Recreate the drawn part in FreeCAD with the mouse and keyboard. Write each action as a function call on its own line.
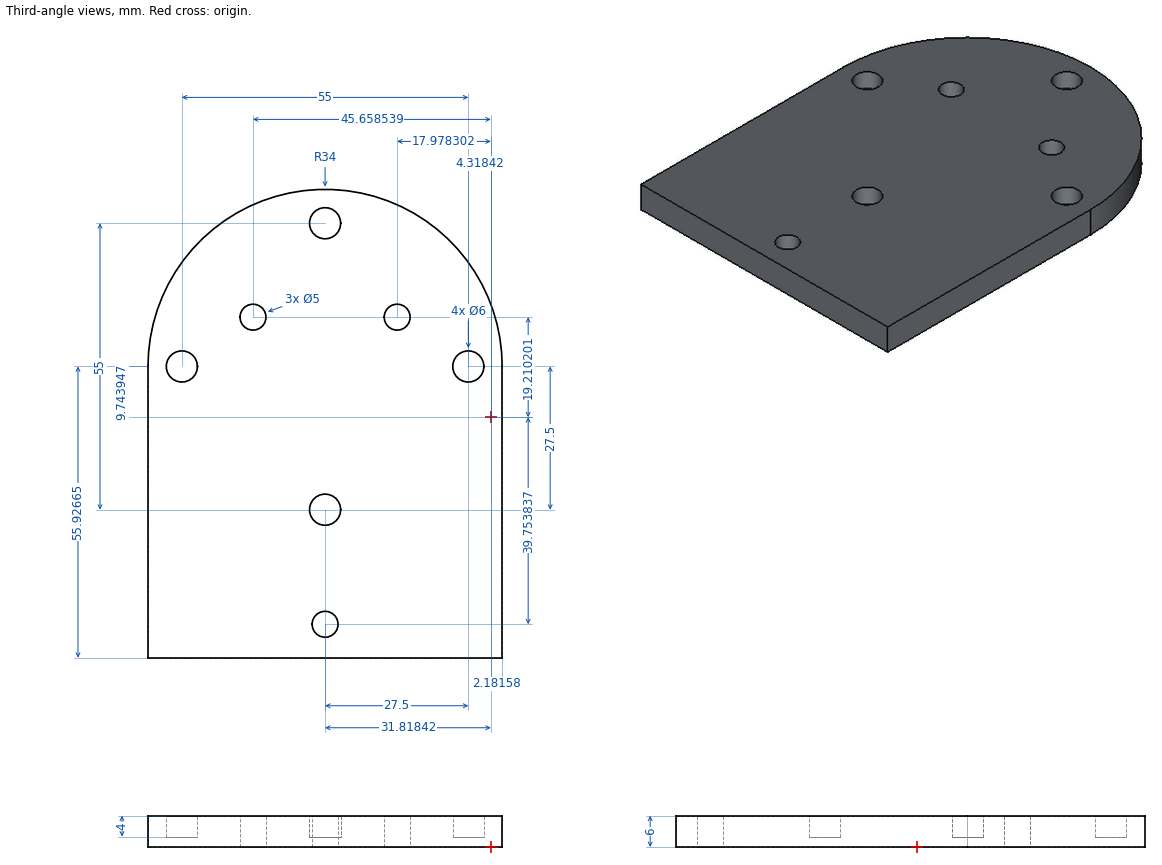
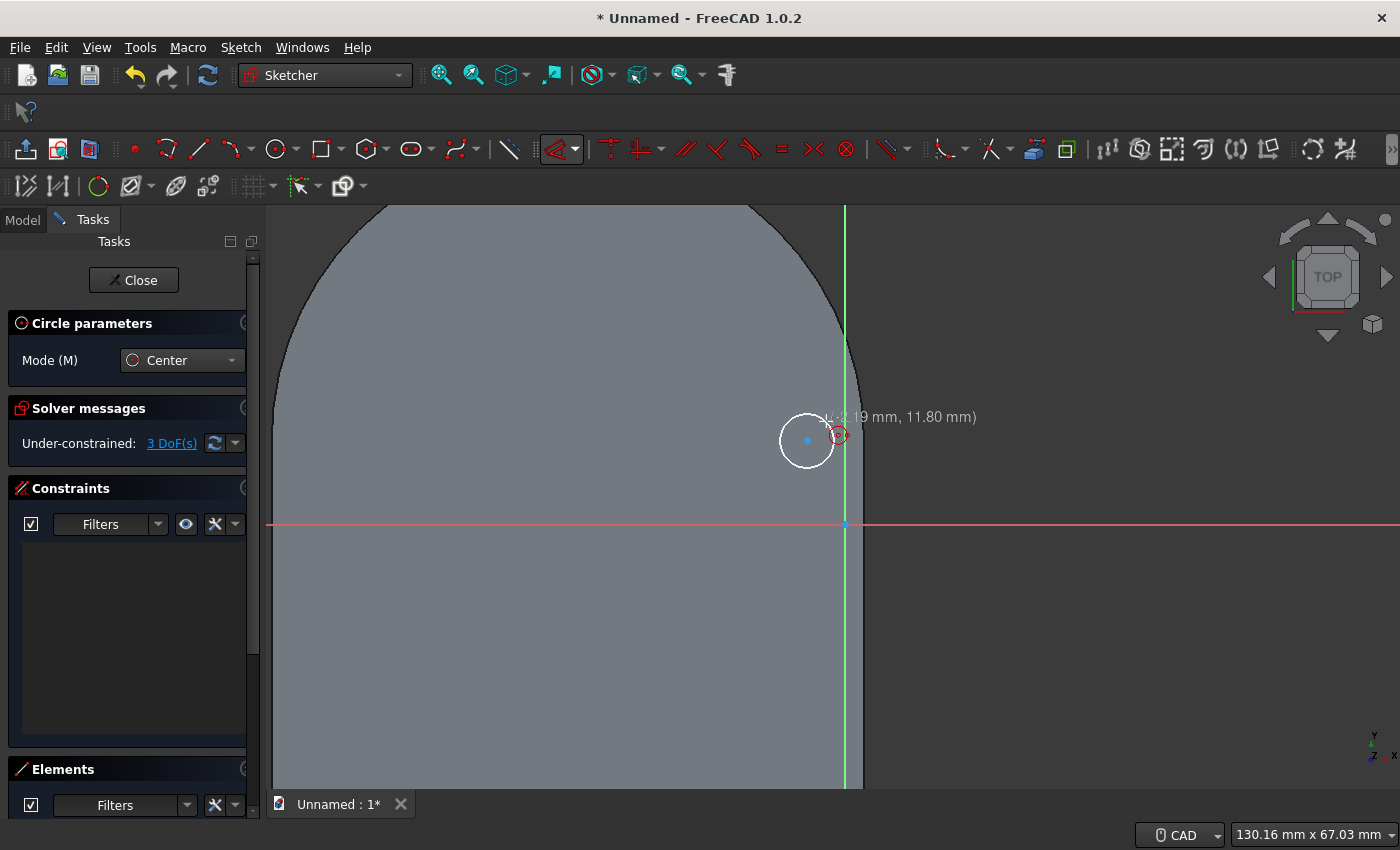
click(568, 680)
click(586, 661)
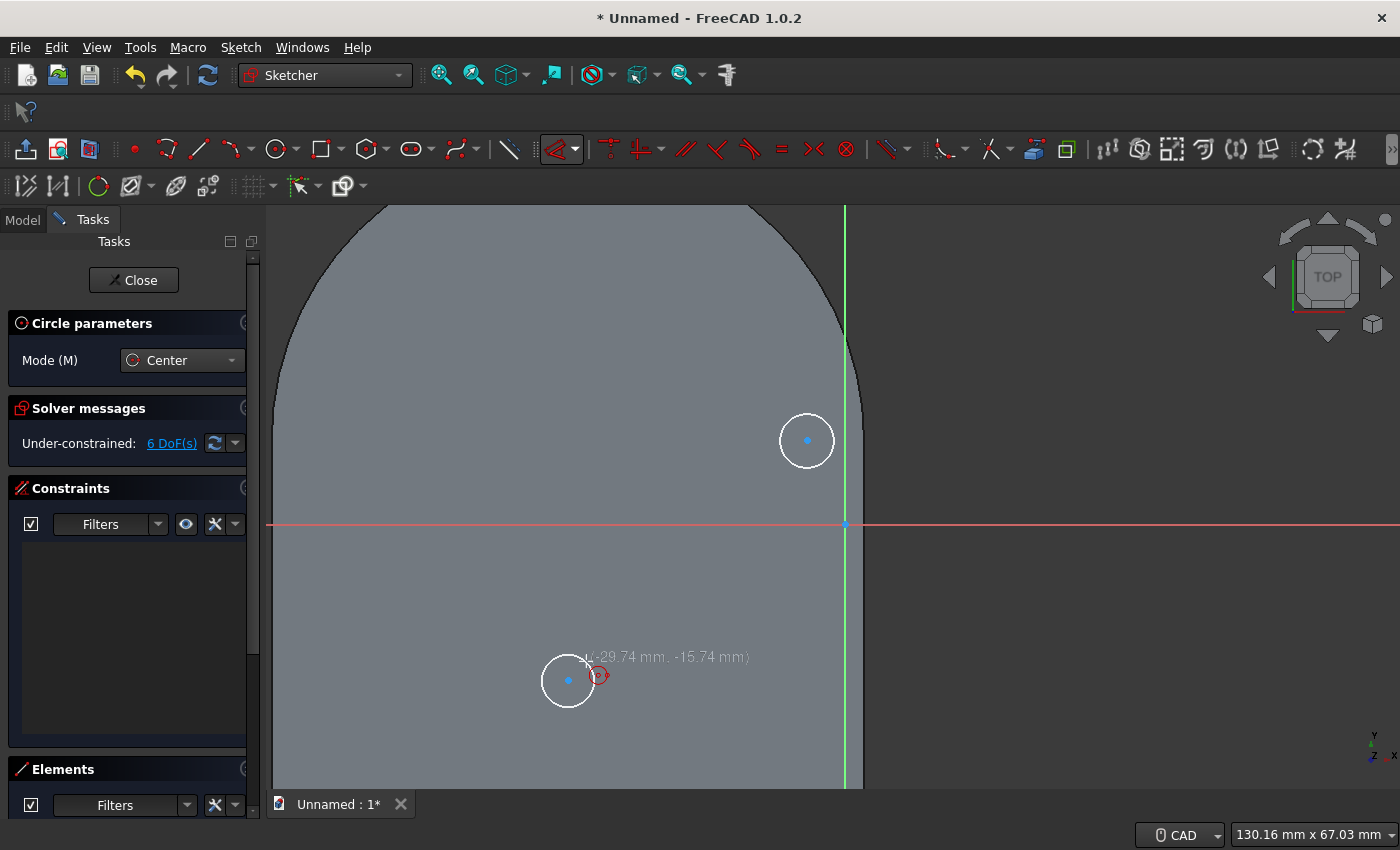
click(328, 440)
click(347, 421)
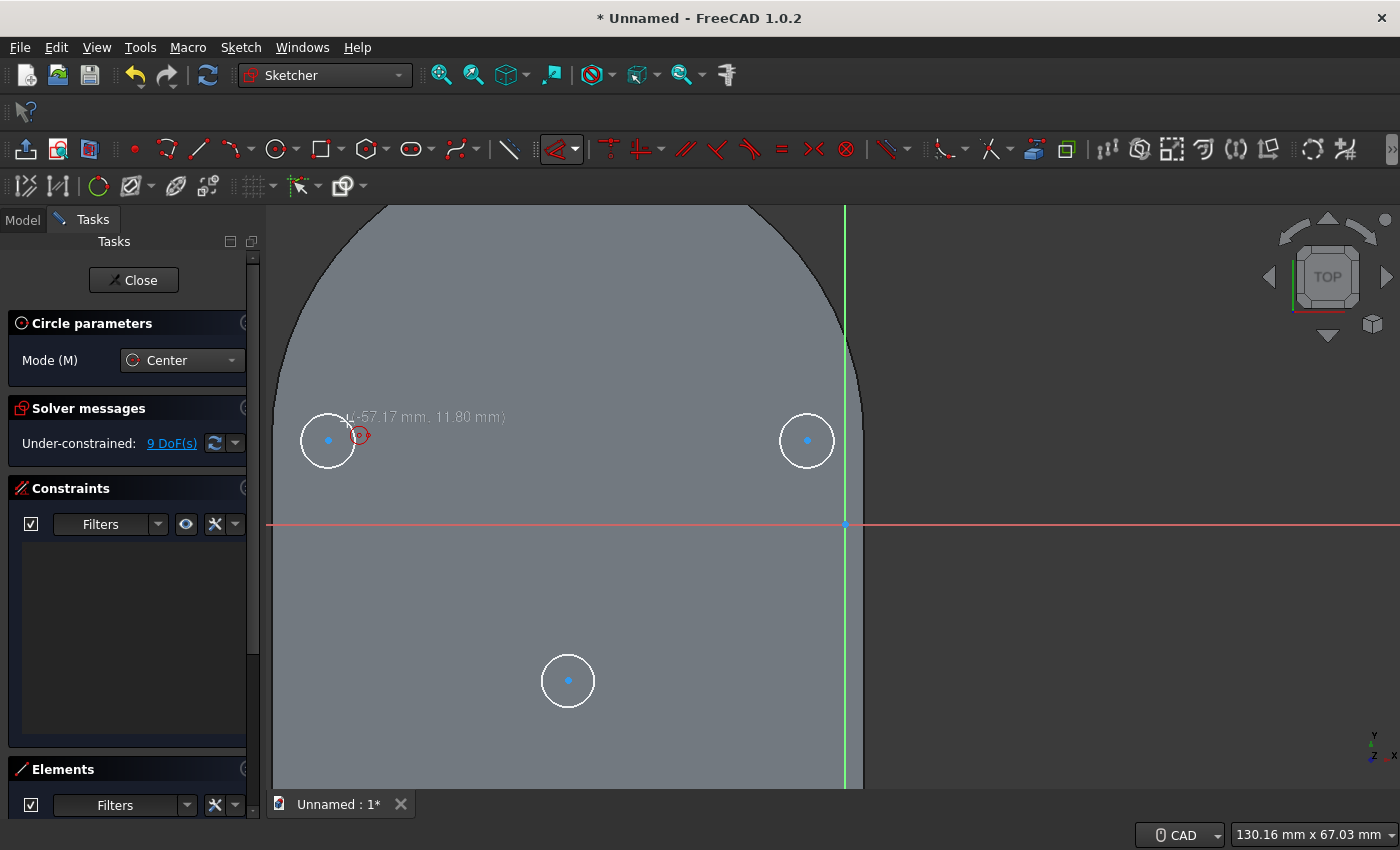
scroll(1153, 613, down, 2)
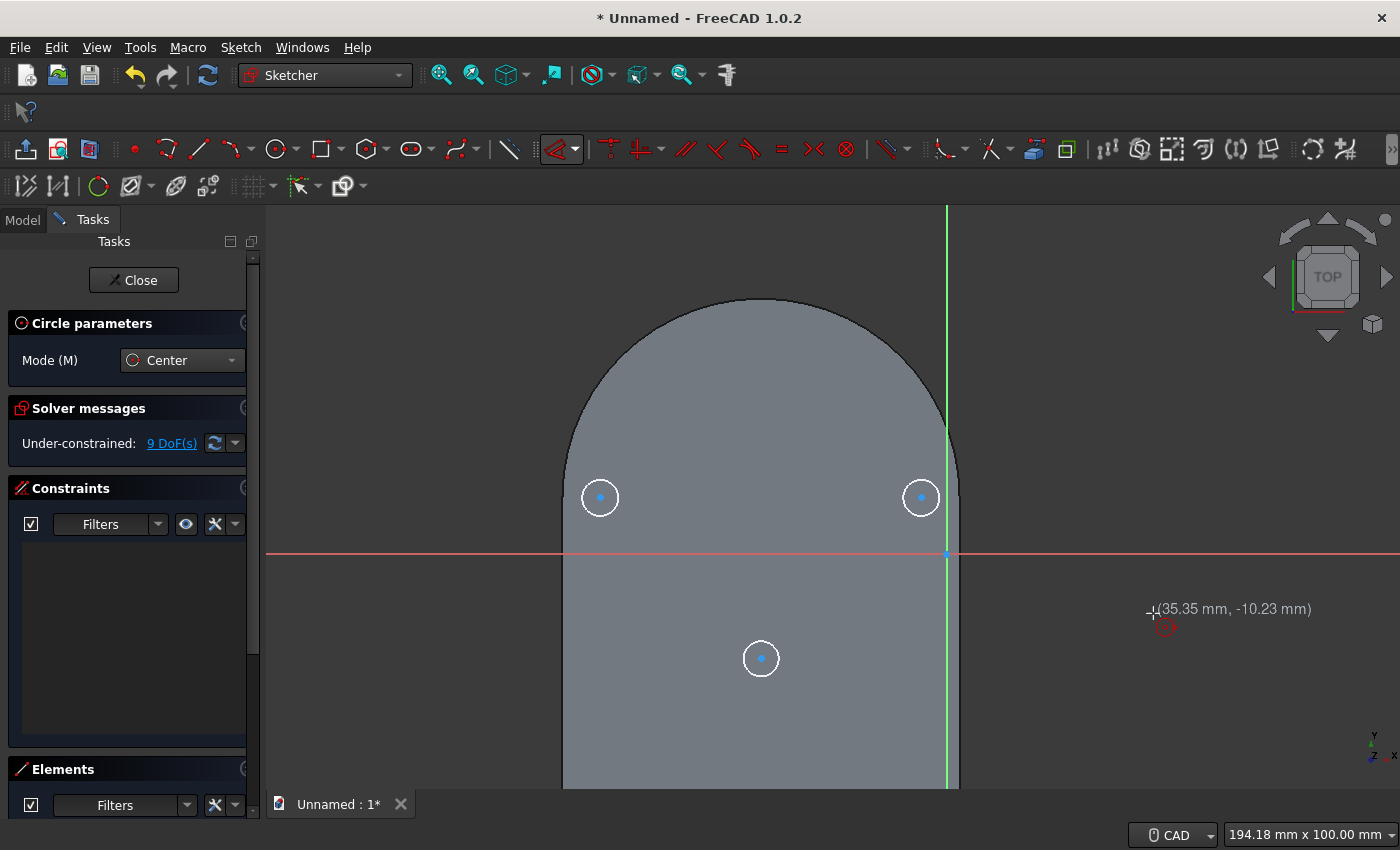
scroll(761, 337, up, 2)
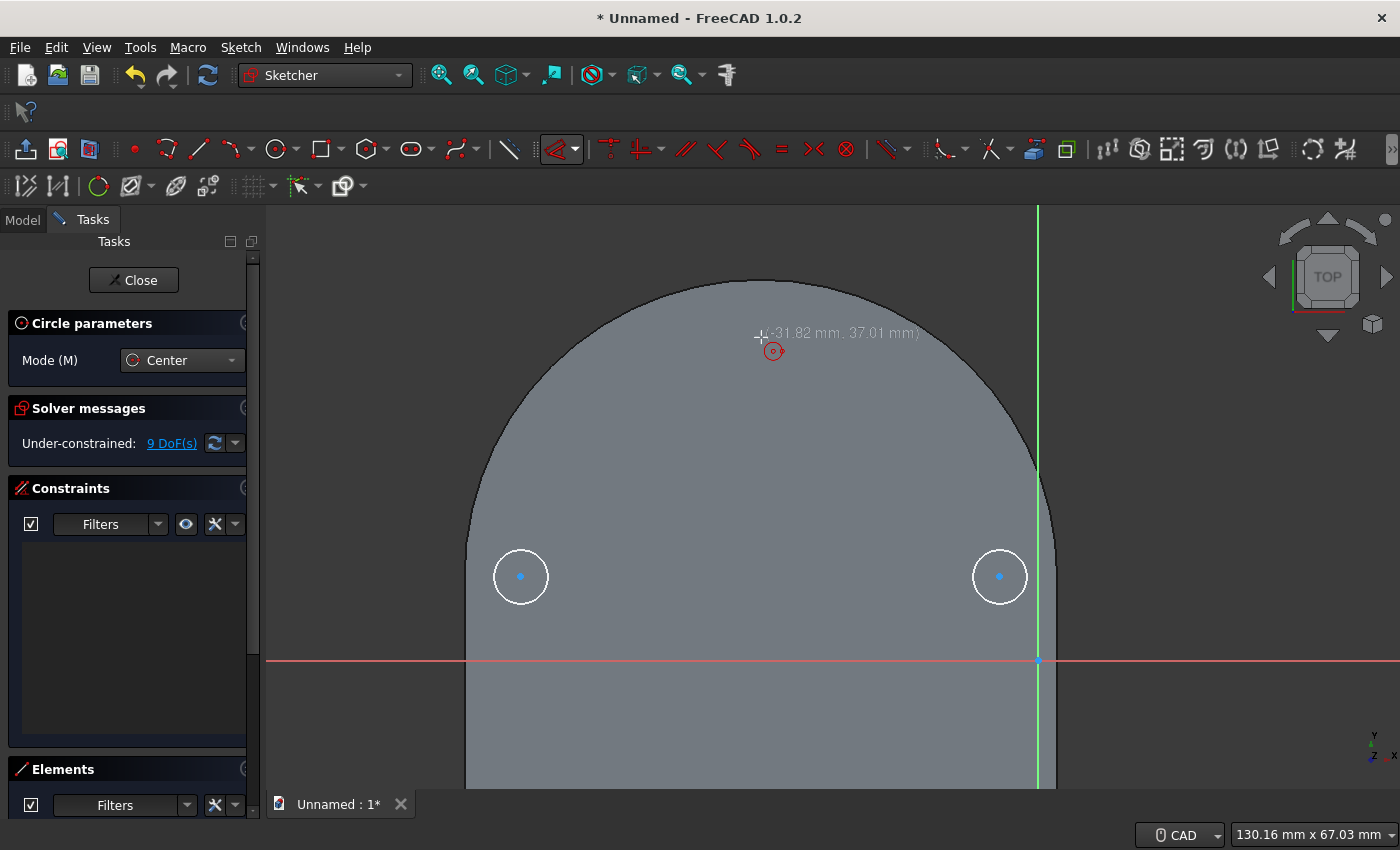
click(761, 336)
click(779, 318)
key(Escape)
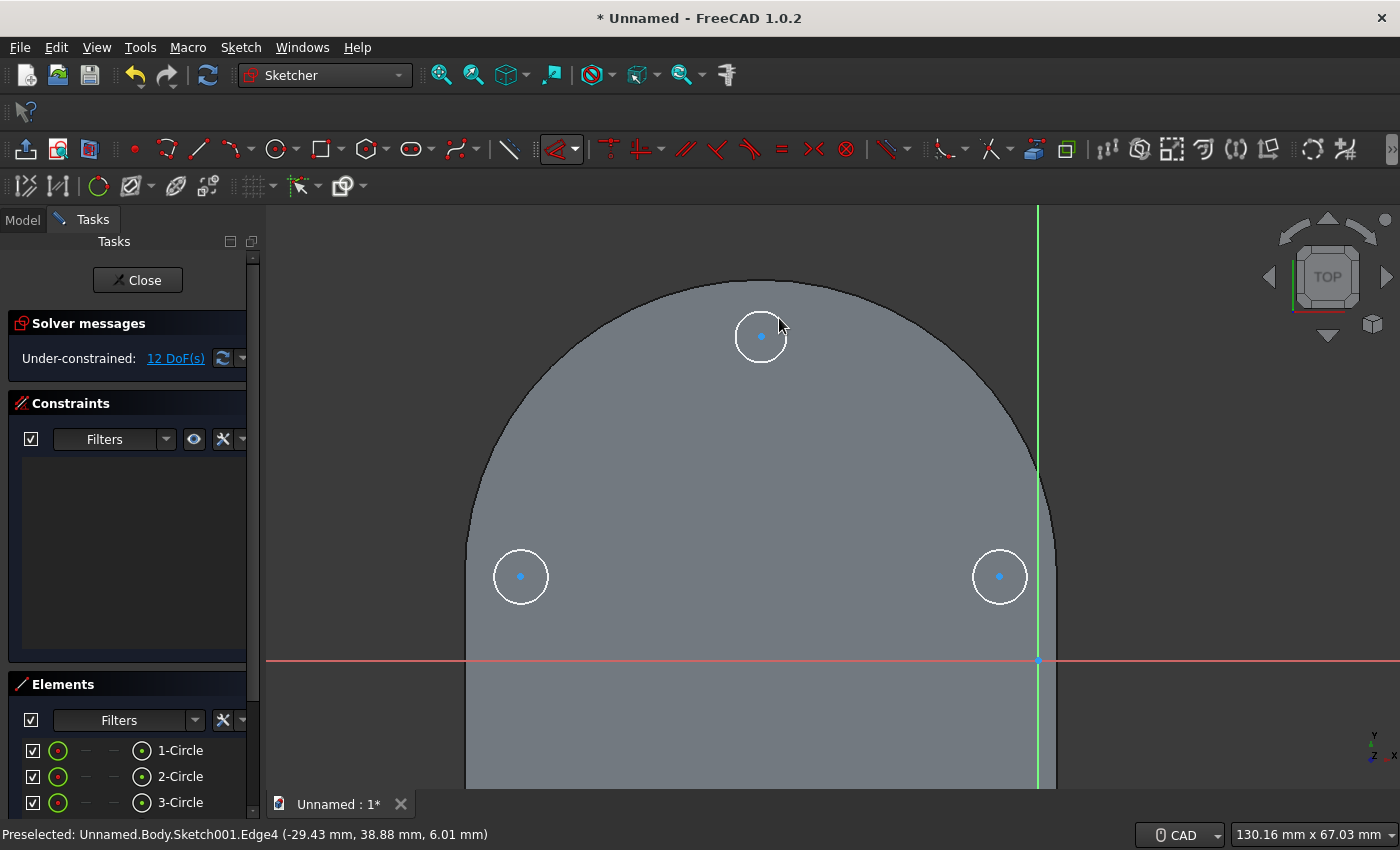
click(1019, 558)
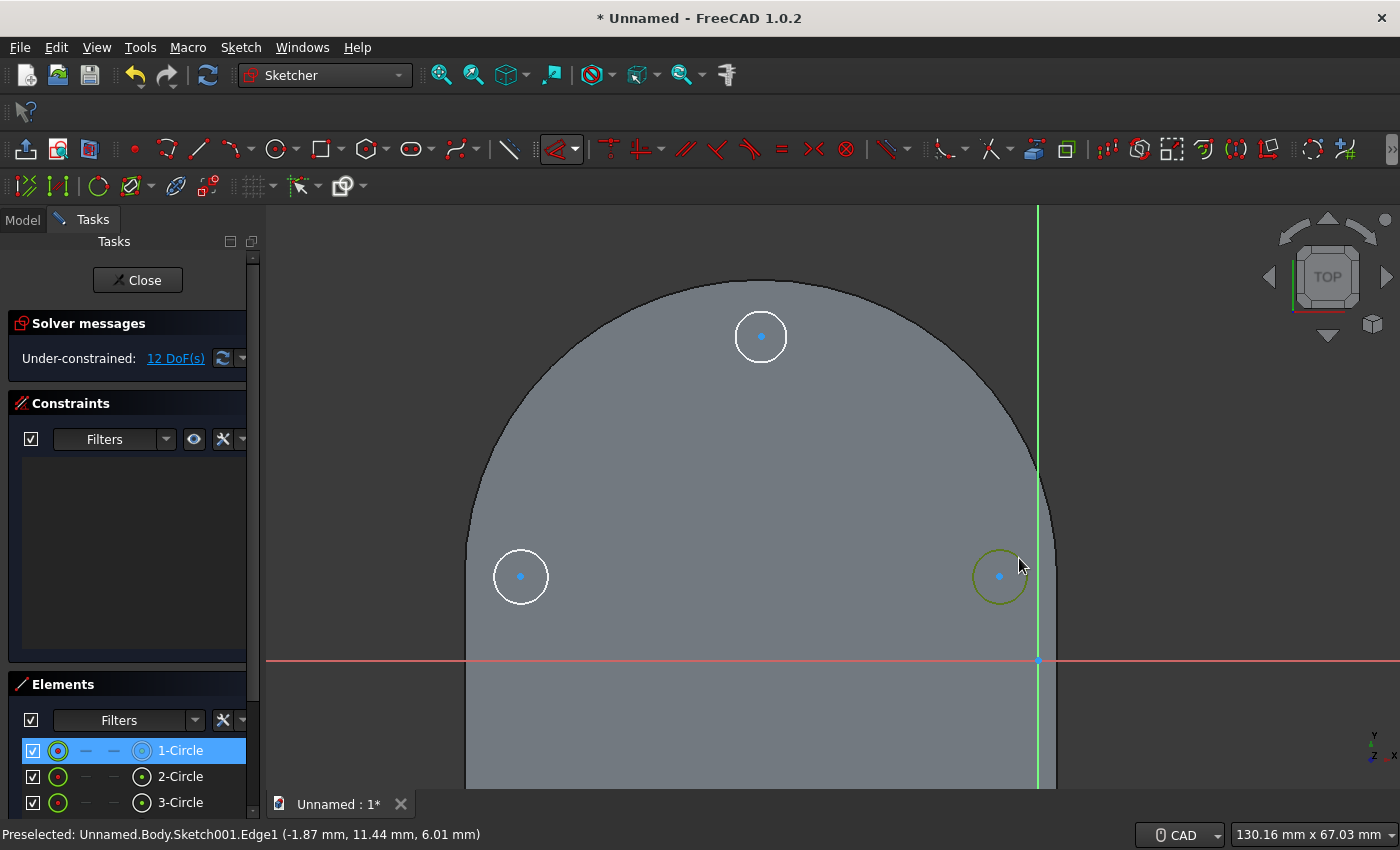
scroll(760, 337, down, 2)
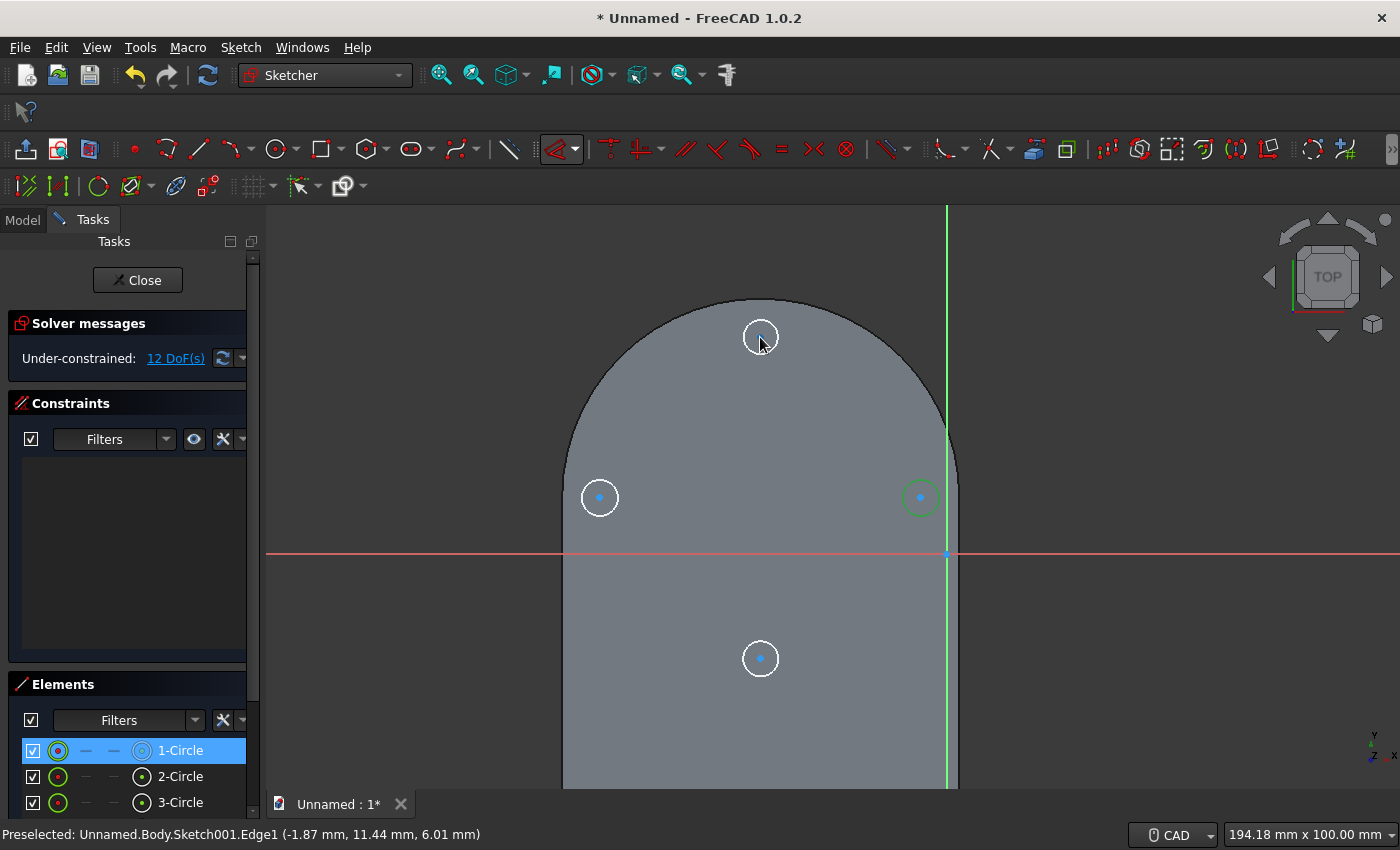
click(773, 646)